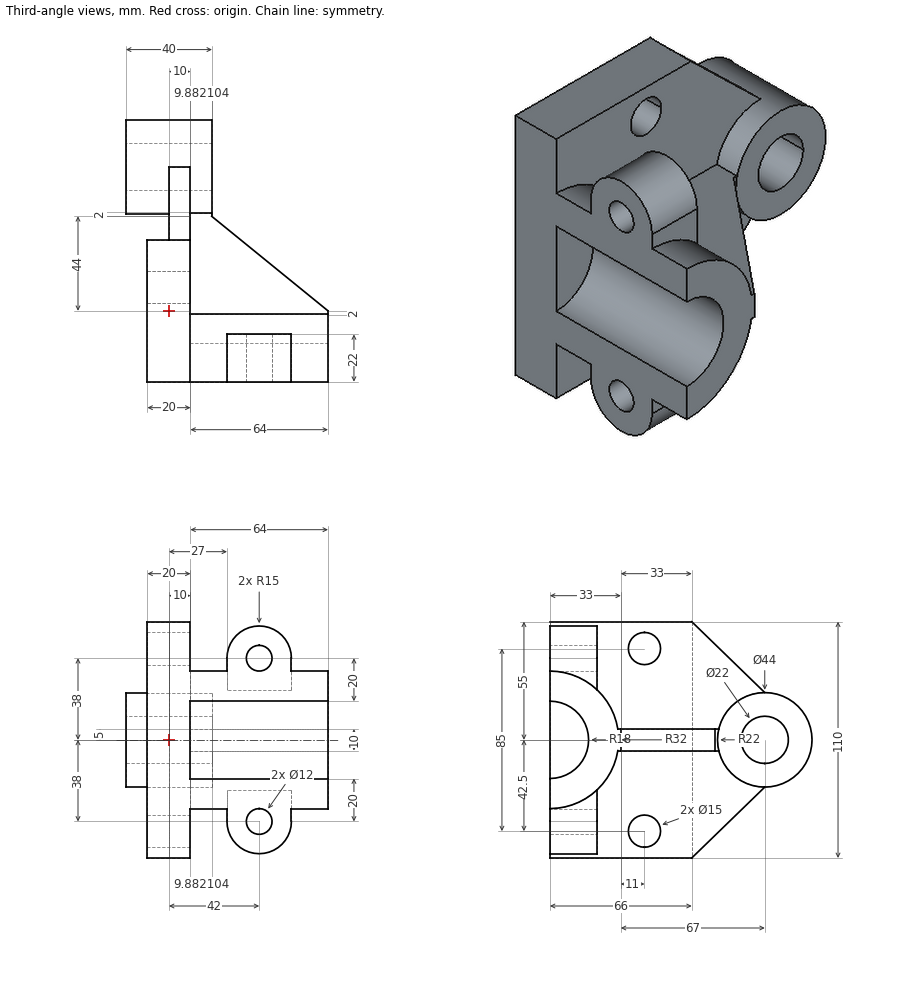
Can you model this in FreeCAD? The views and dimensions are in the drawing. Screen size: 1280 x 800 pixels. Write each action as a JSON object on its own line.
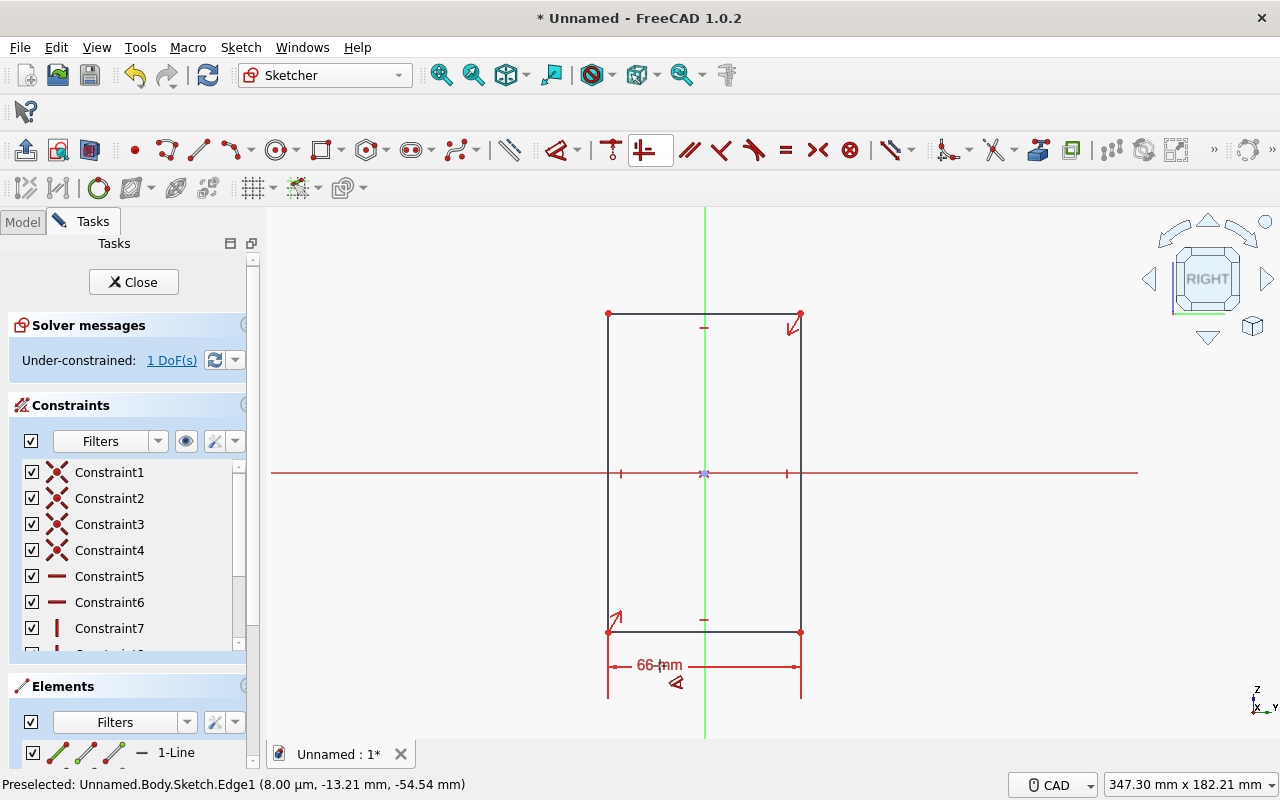
{"action": "left_click", "coordinate": [801, 537]}
{"action": "left_click", "coordinate": [835, 400]}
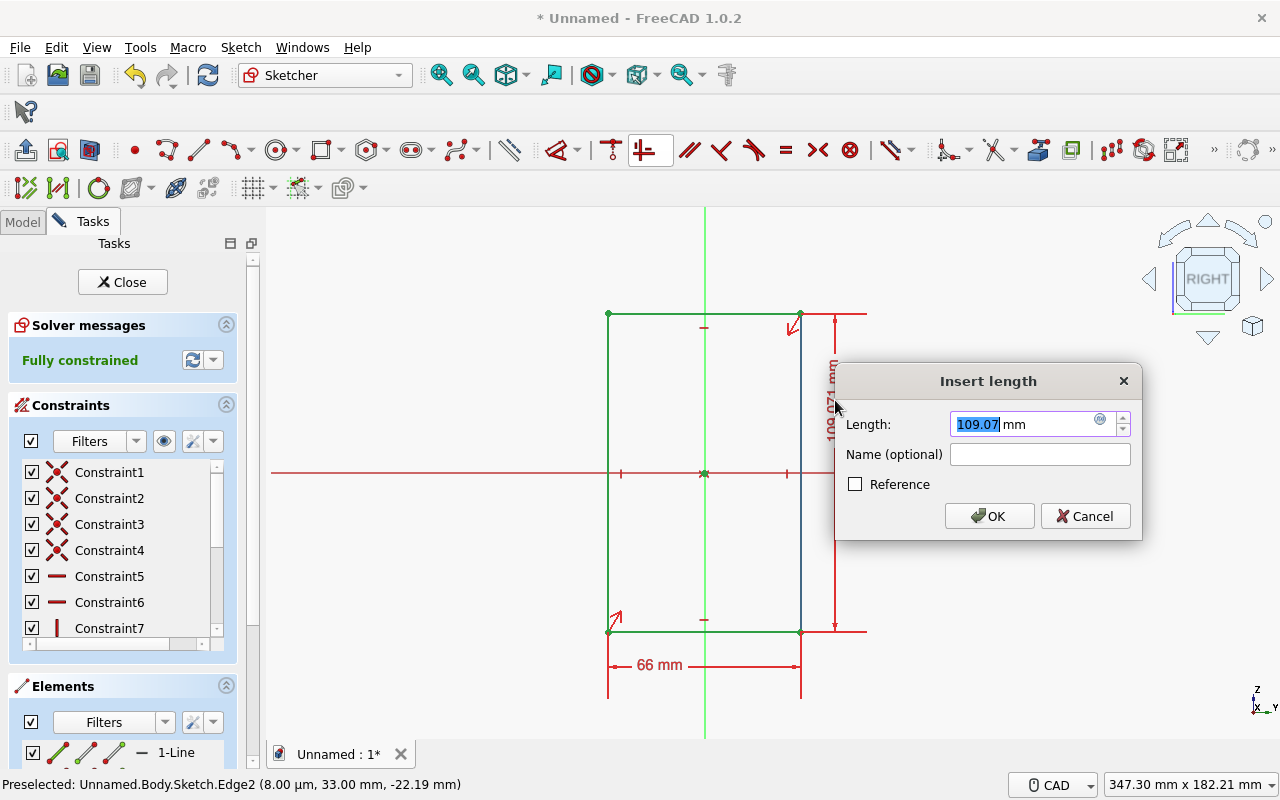
{"action": "type", "text": "110"}
{"action": "key", "text": "Return"}
{"action": "key", "text": "Escape"}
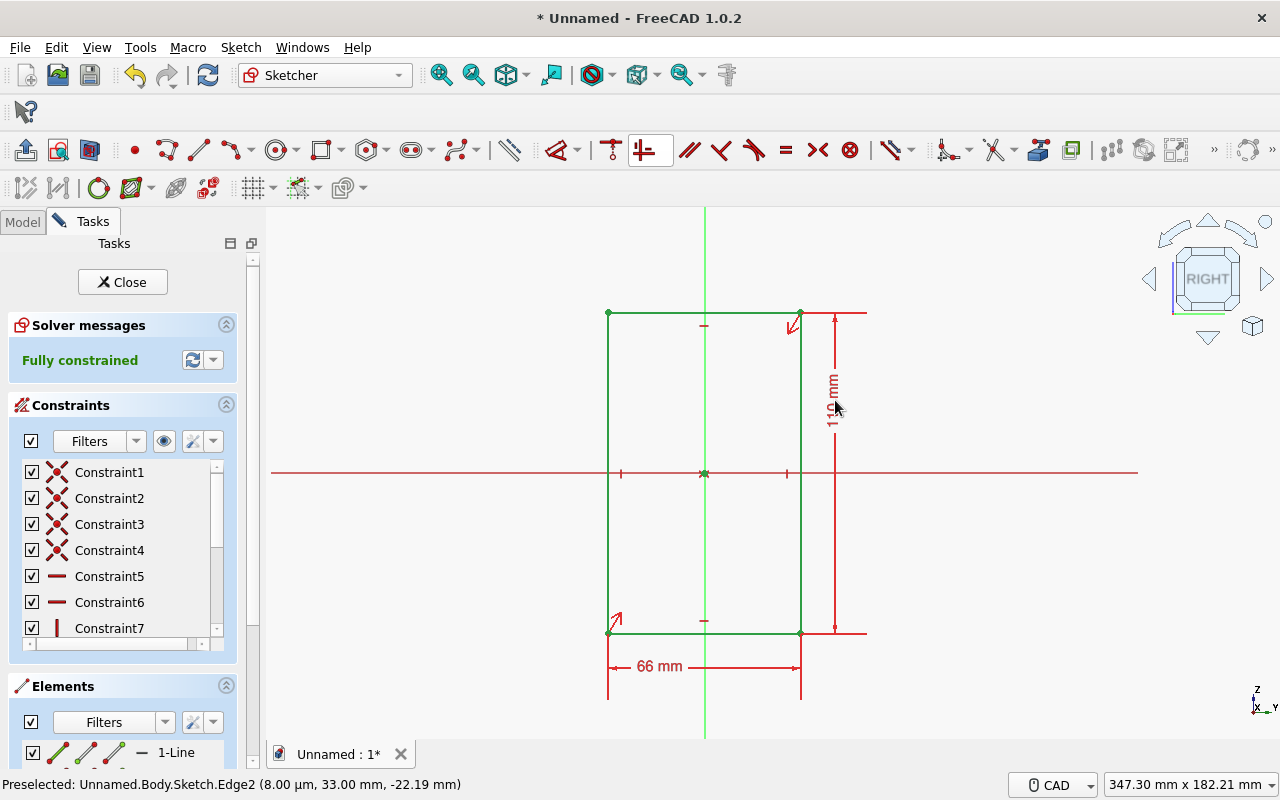
{"action": "left_click", "coordinate": [123, 282]}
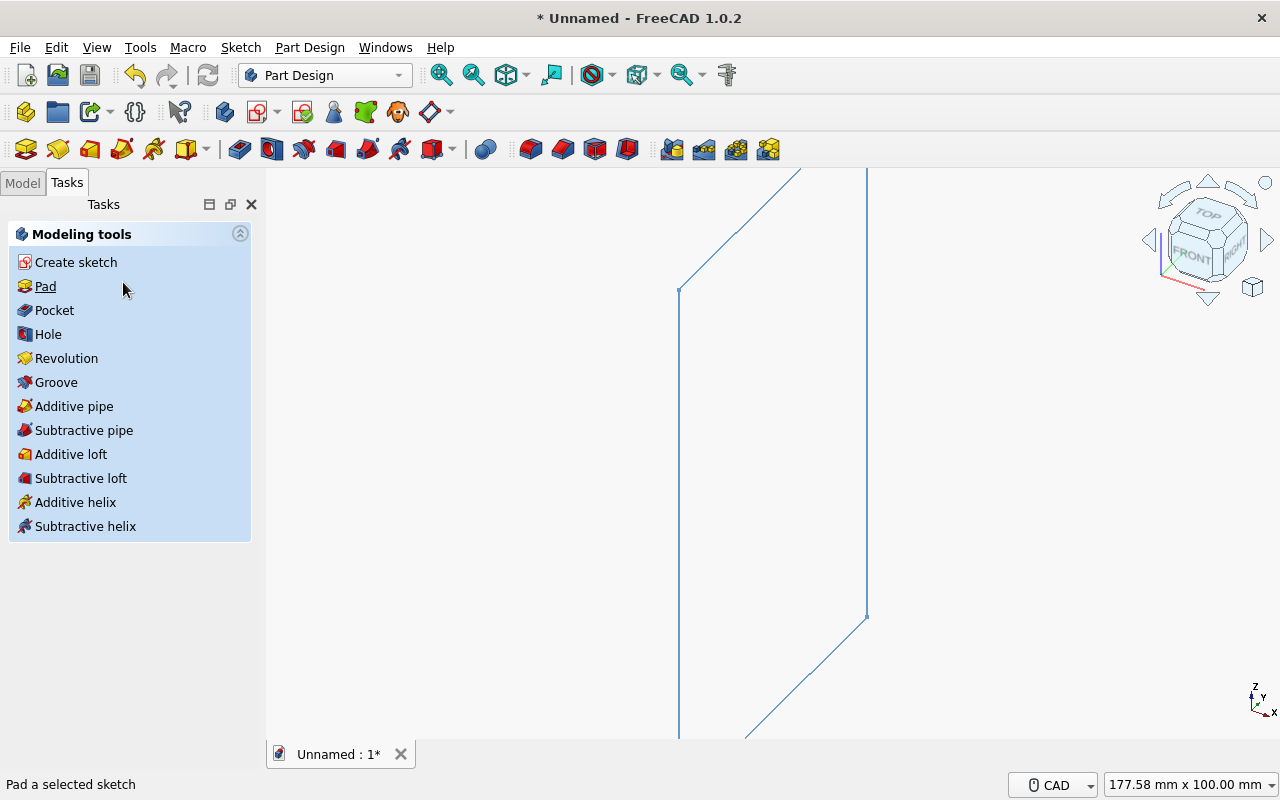
{"action": "left_click", "coordinate": [26, 150]}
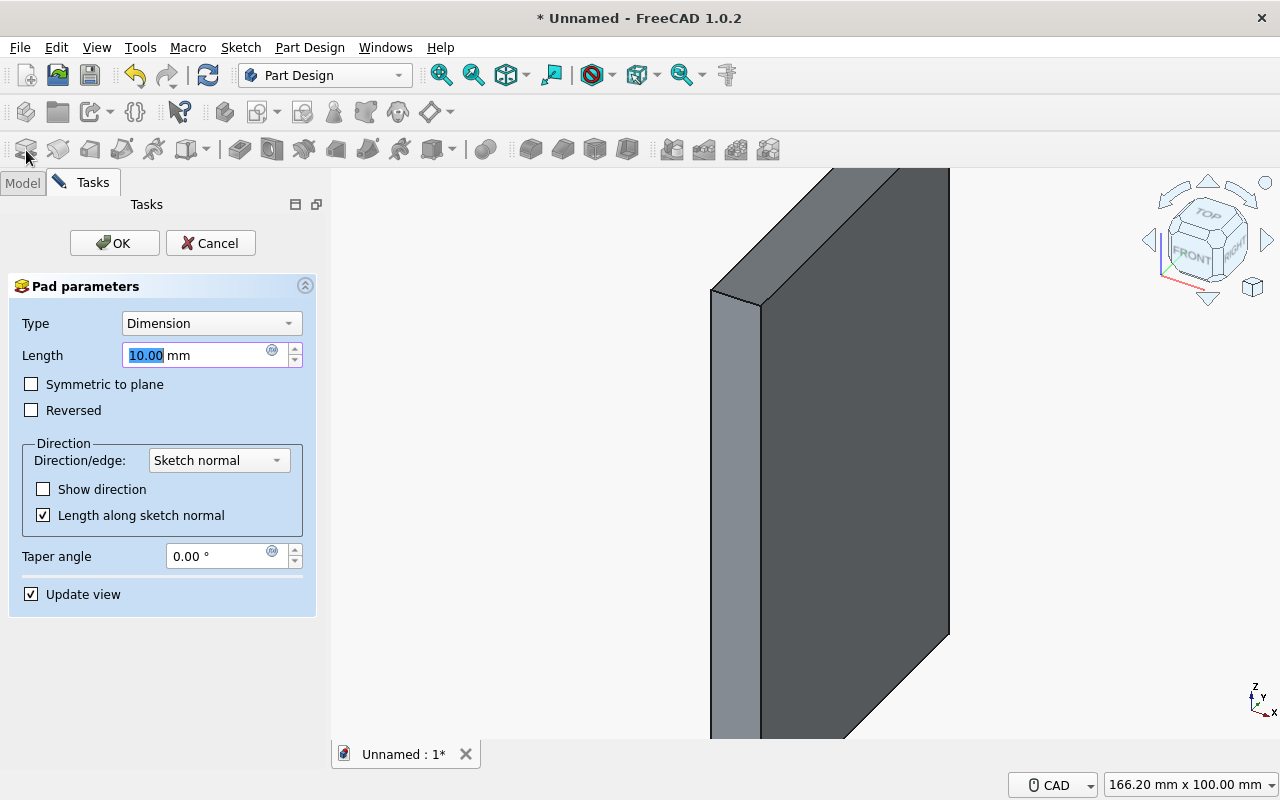
{"action": "type", "text": "20"}
{"action": "key", "text": "Tab"}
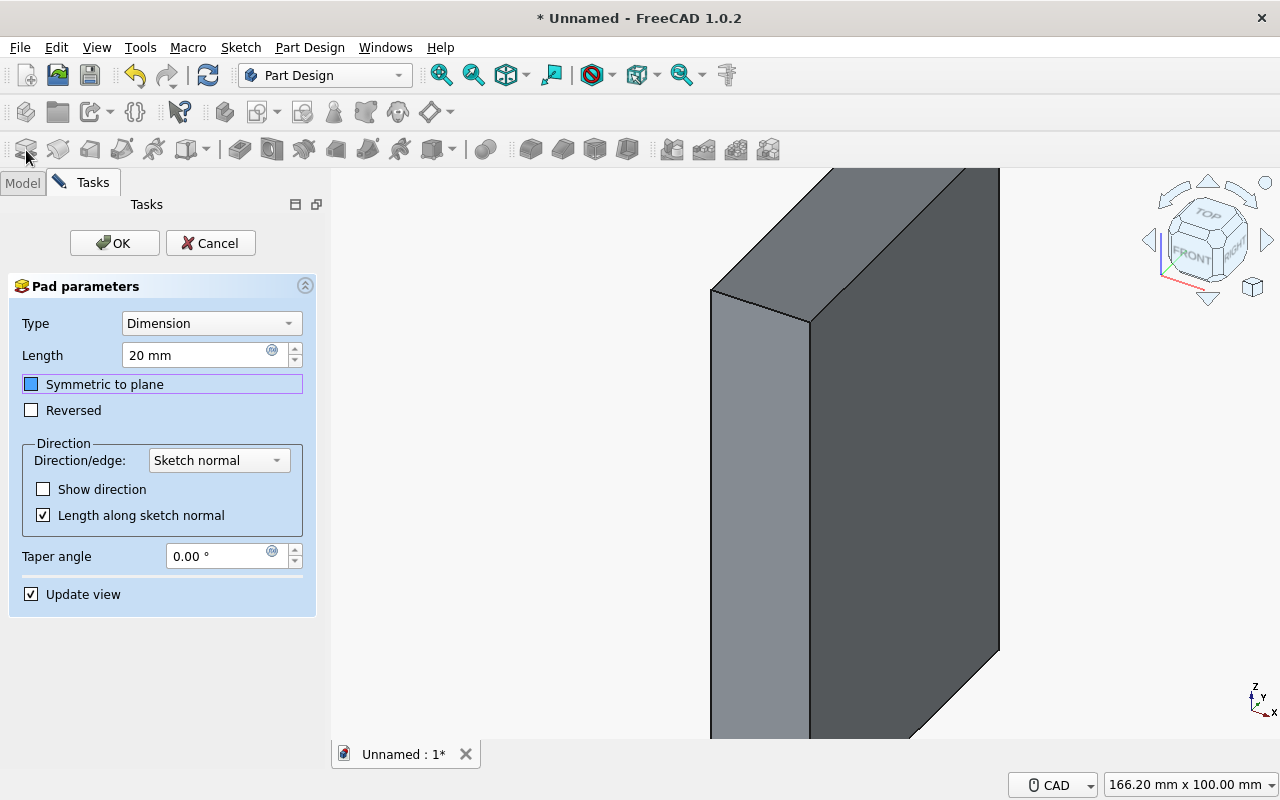
{"action": "left_click", "coordinate": [30, 384]}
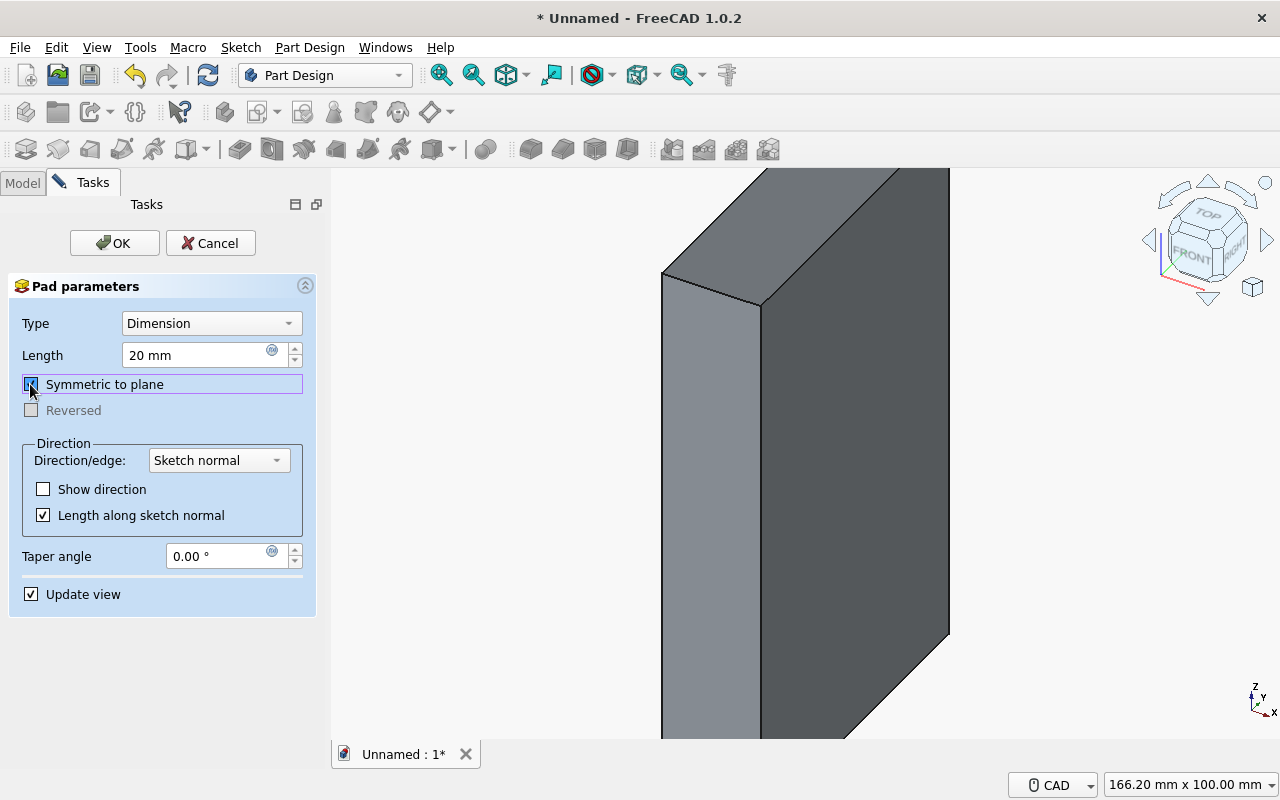
{"action": "left_click", "coordinate": [115, 243]}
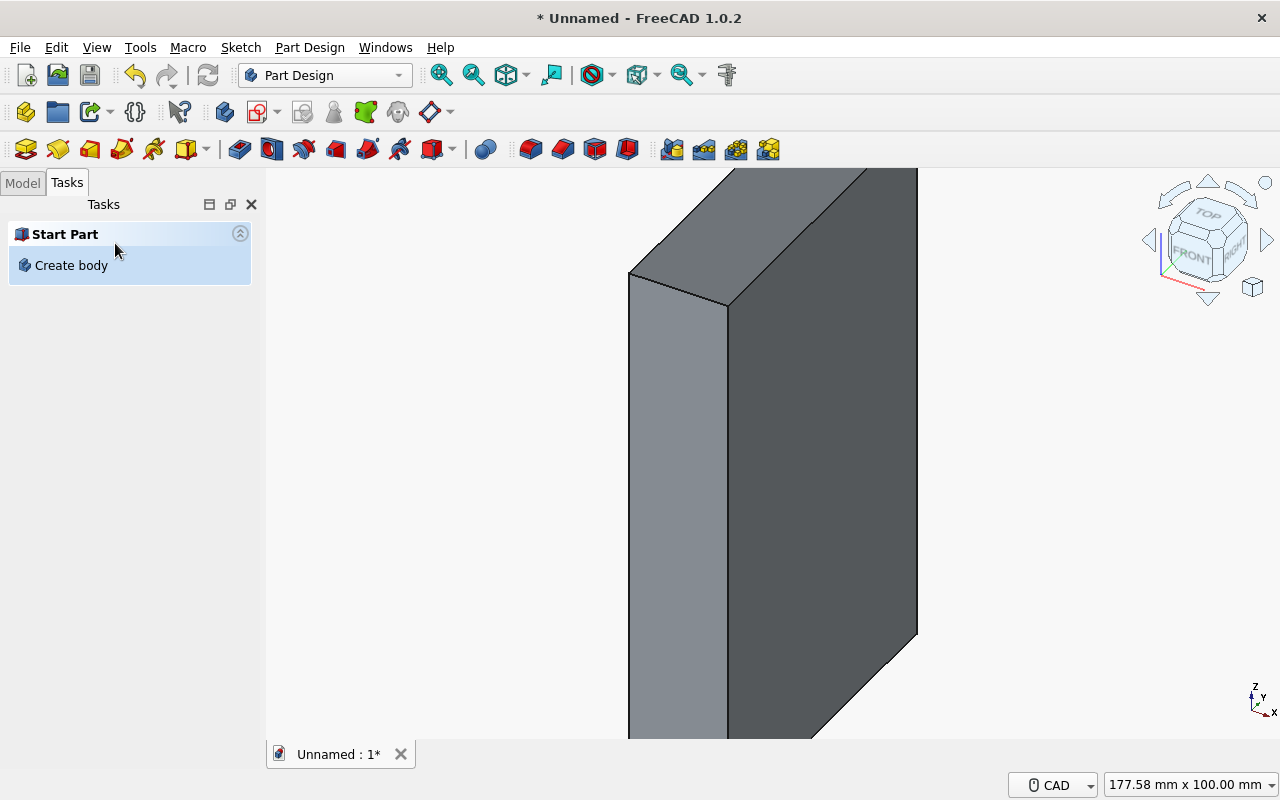
{"action": "left_click", "coordinate": [442, 76]}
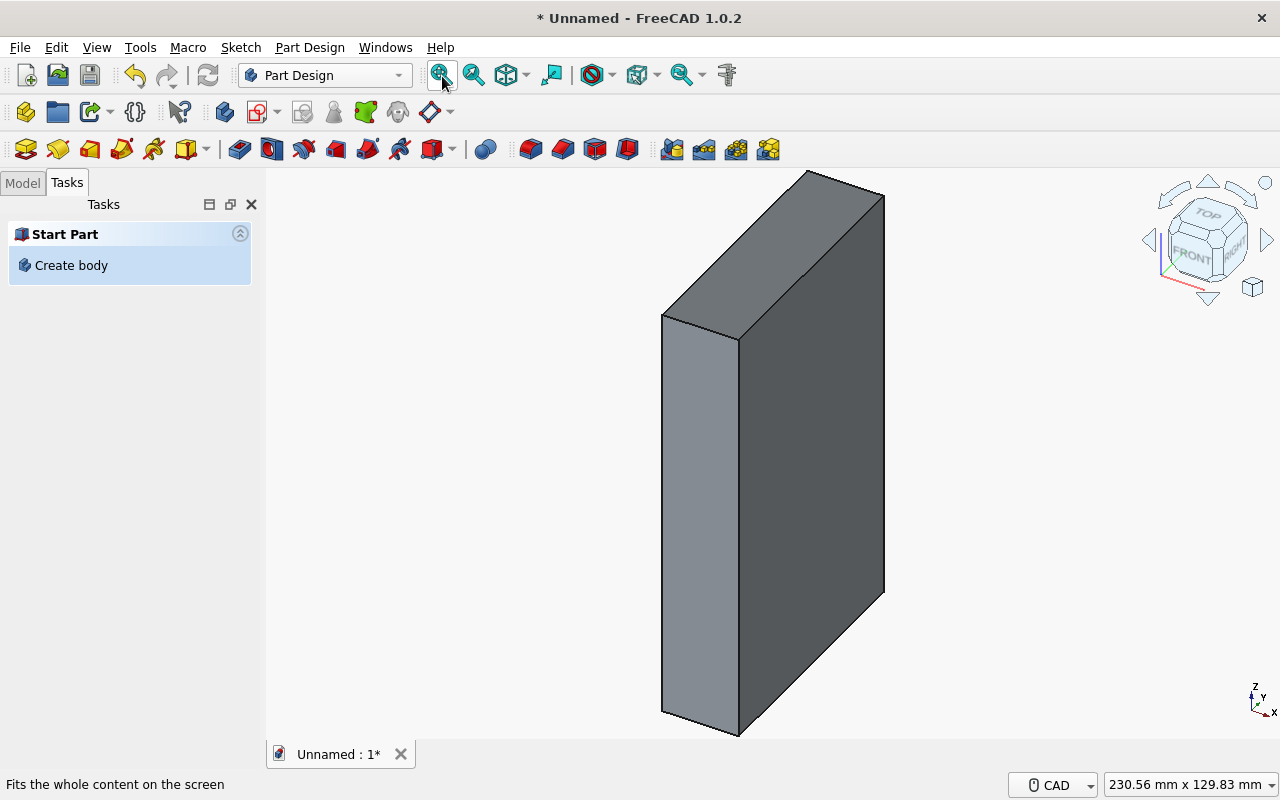
{"action": "left_click", "coordinate": [811, 465]}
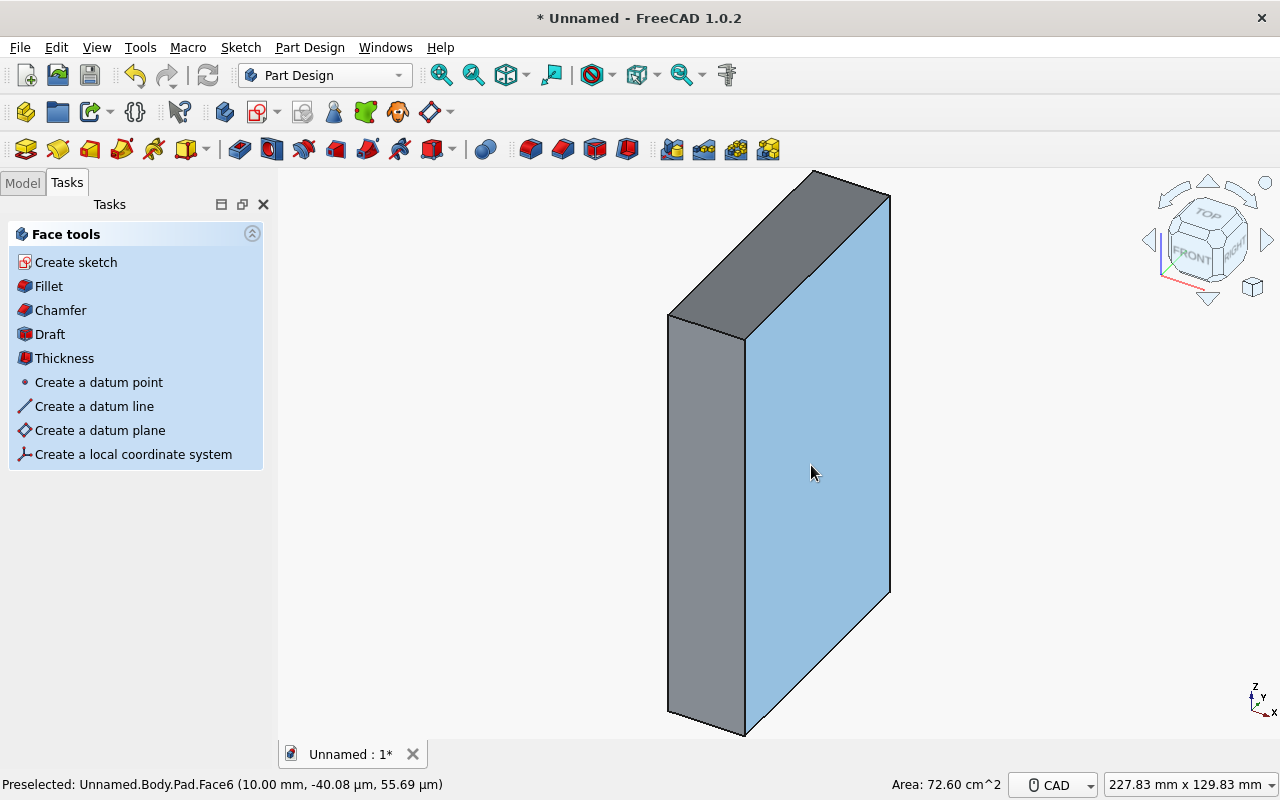
{"action": "left_click", "coordinate": [258, 112]}